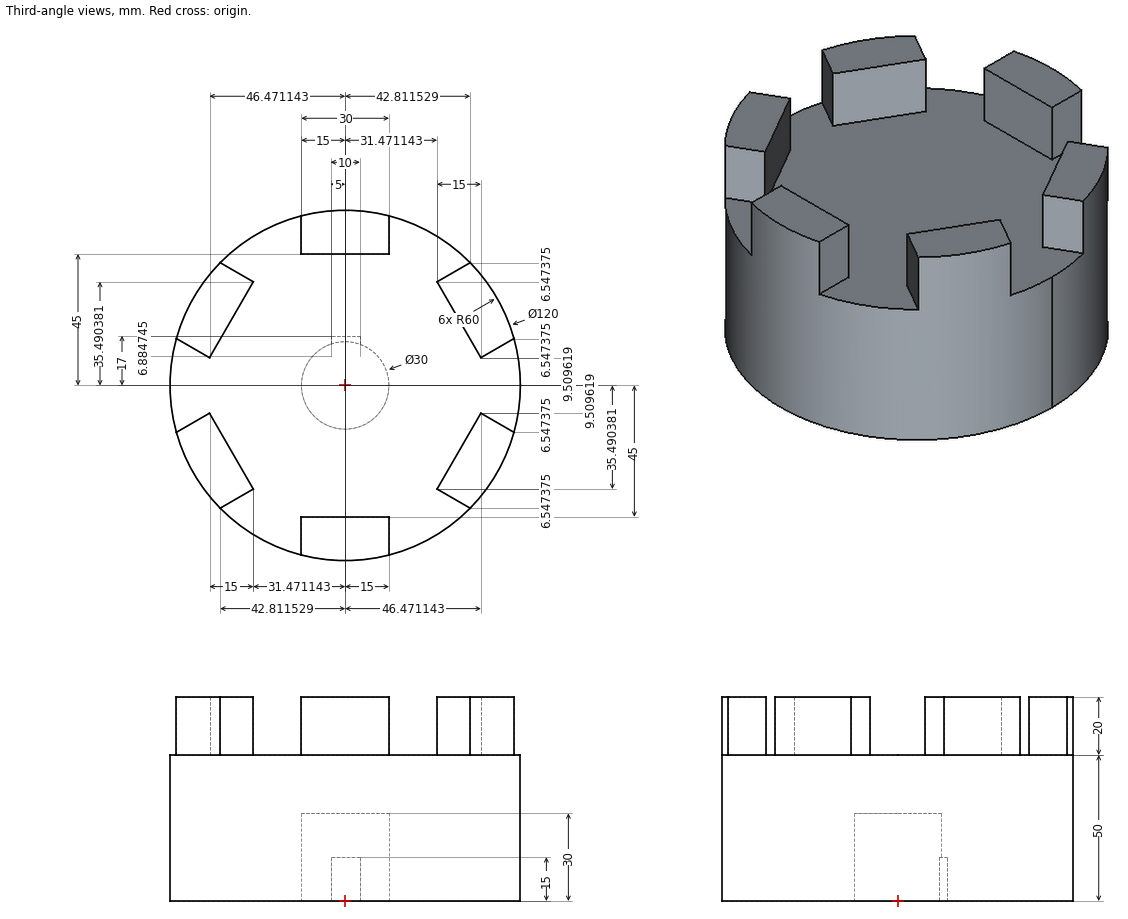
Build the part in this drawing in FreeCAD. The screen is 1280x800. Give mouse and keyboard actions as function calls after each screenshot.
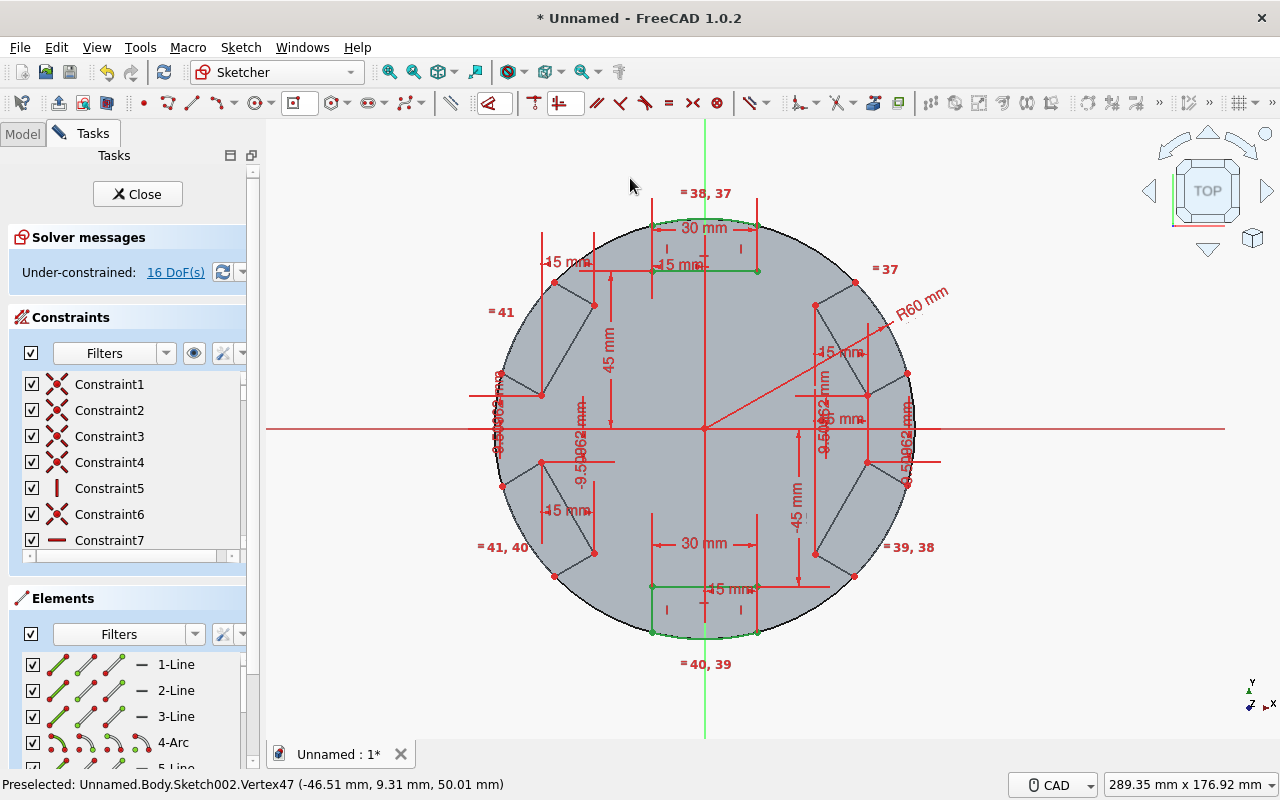
scroll(844, 290, up, 3)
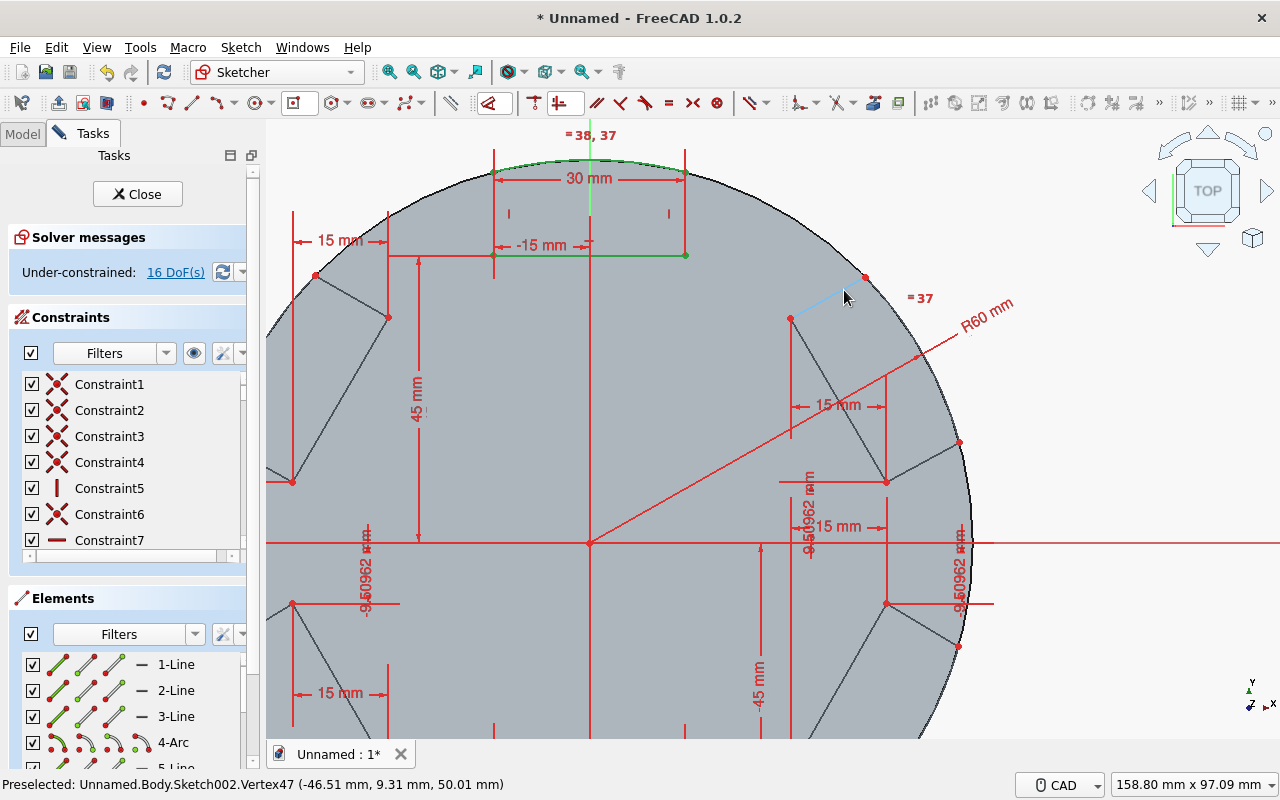
click(843, 290)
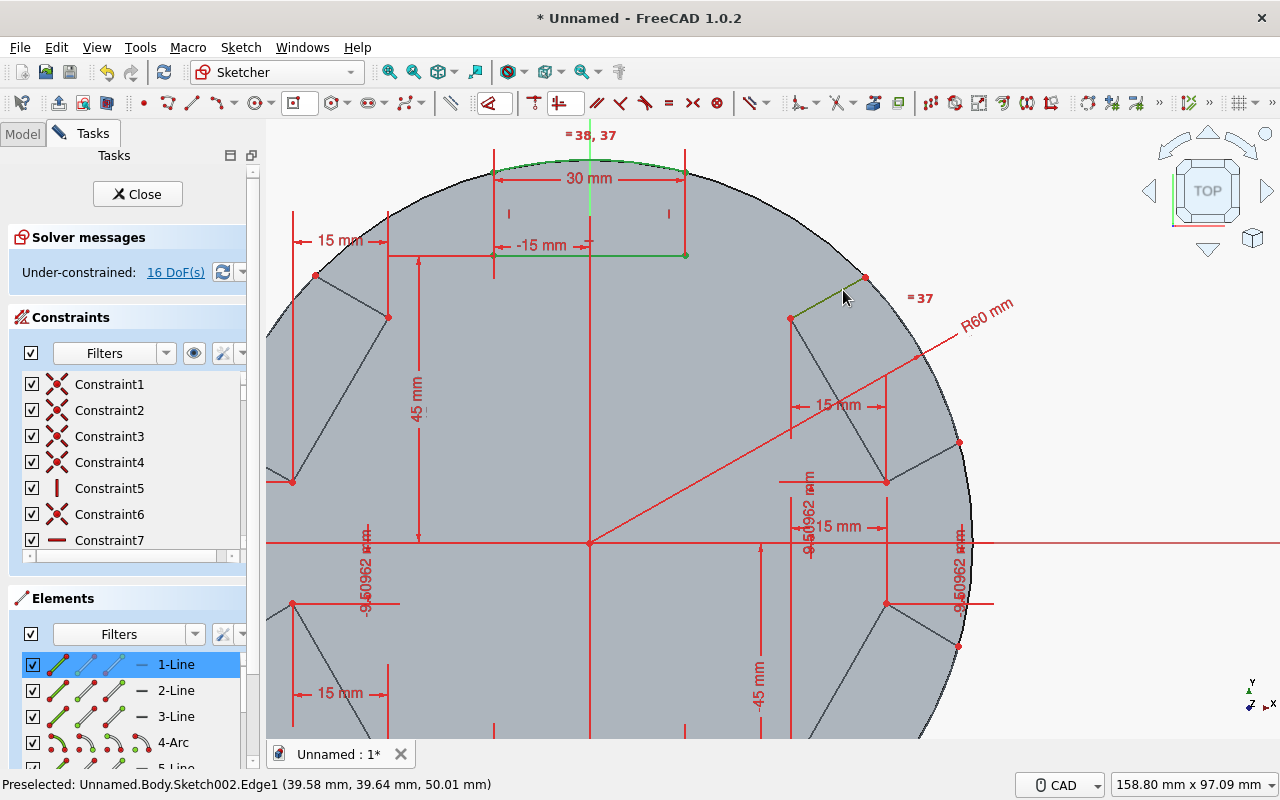
key(i)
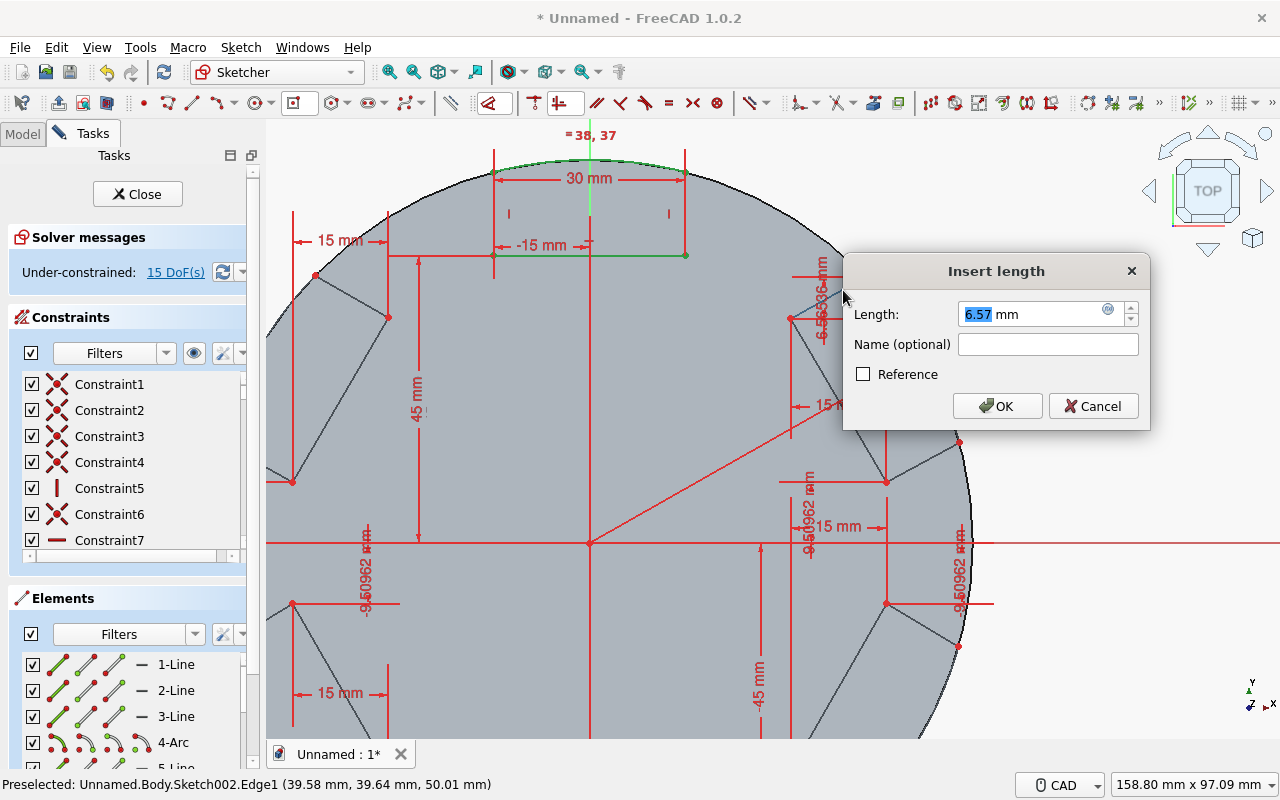
text(6.547375)
key(Return)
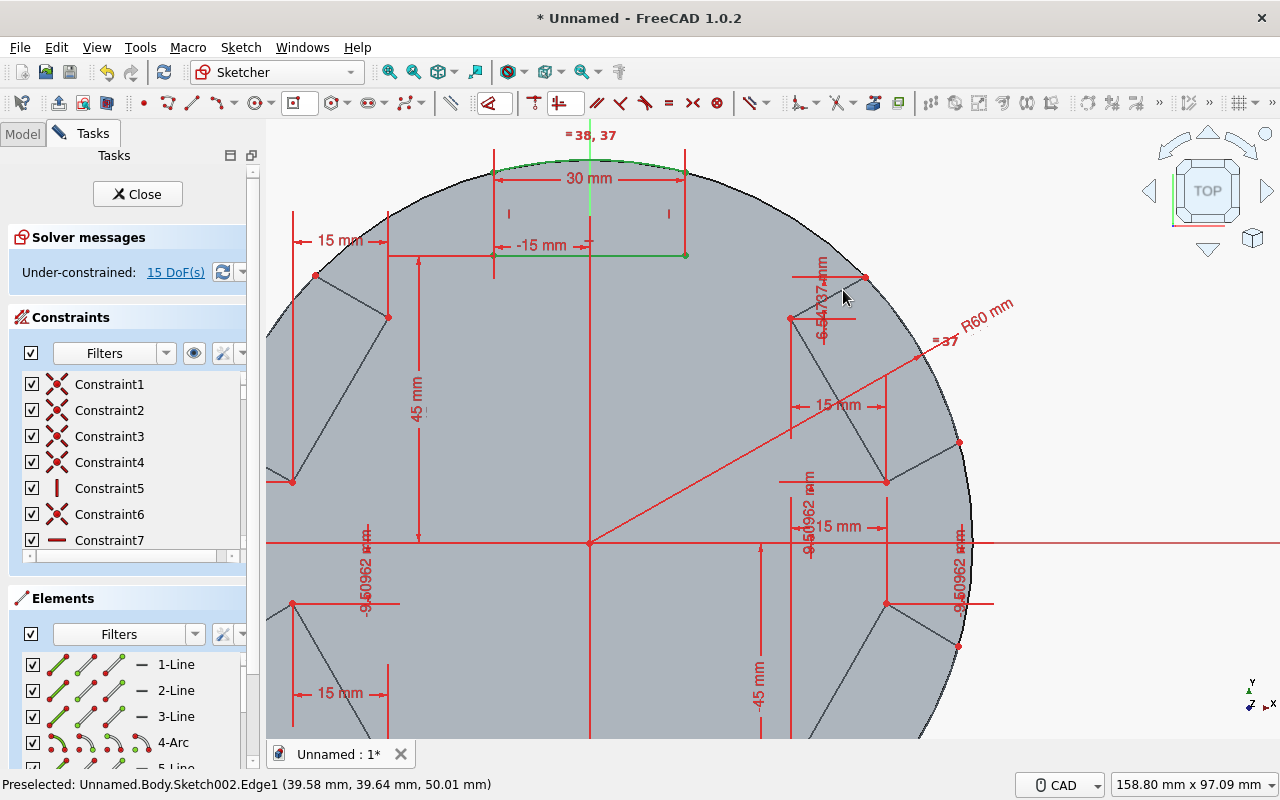
click(908, 470)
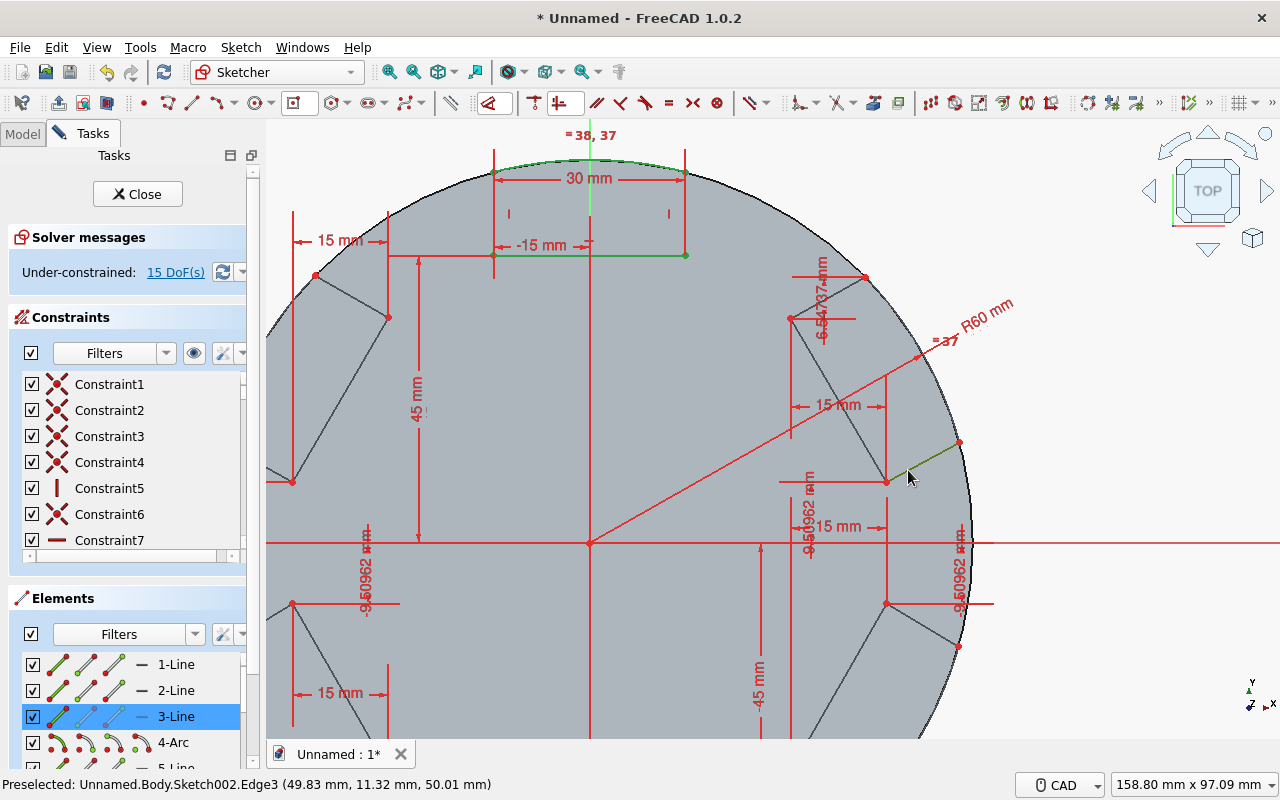
key(i)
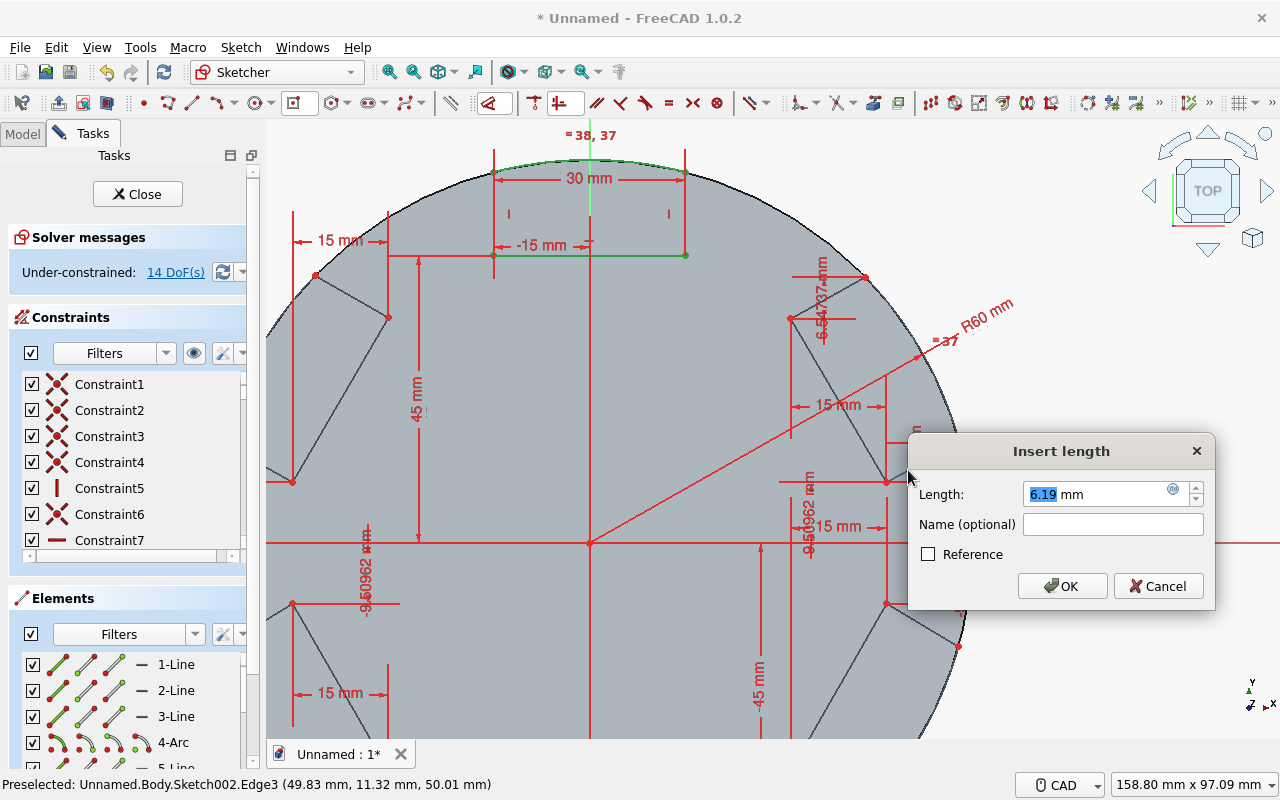
text(6.547375)
key(Return)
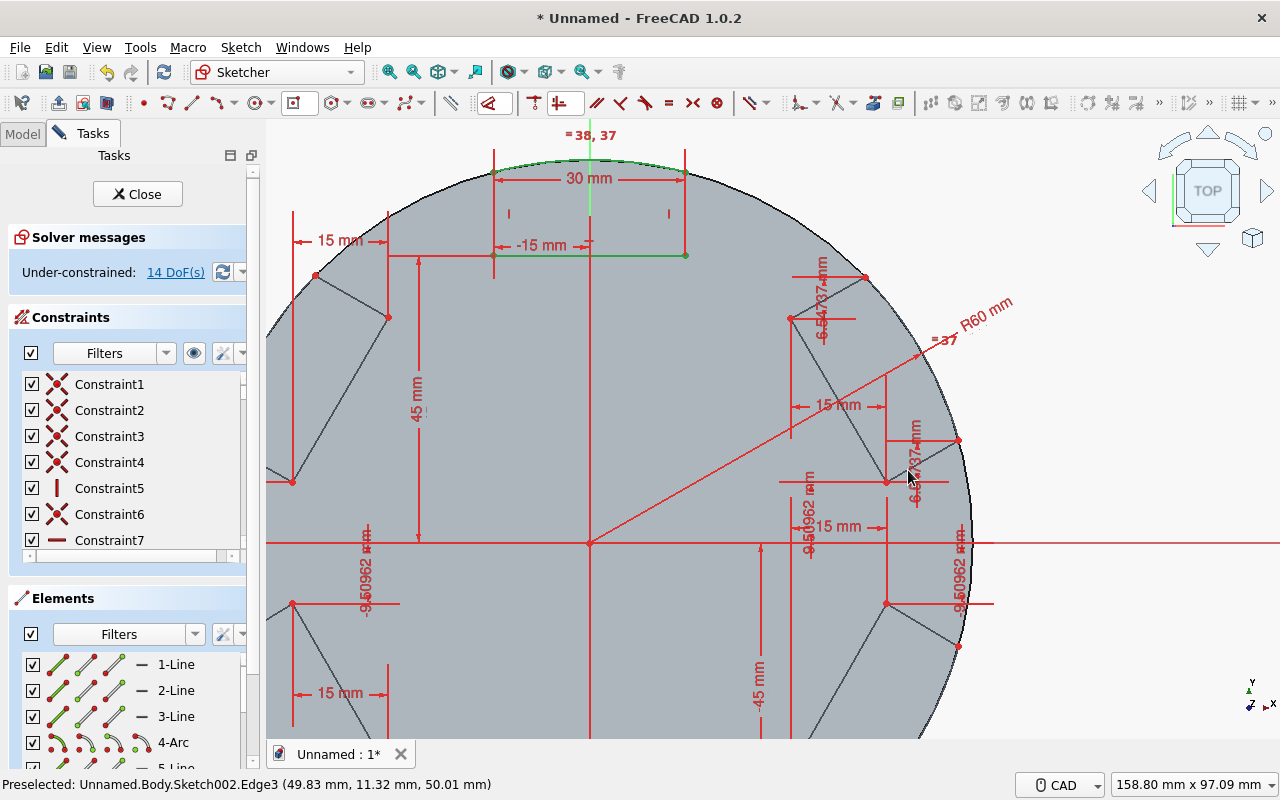
click(937, 634)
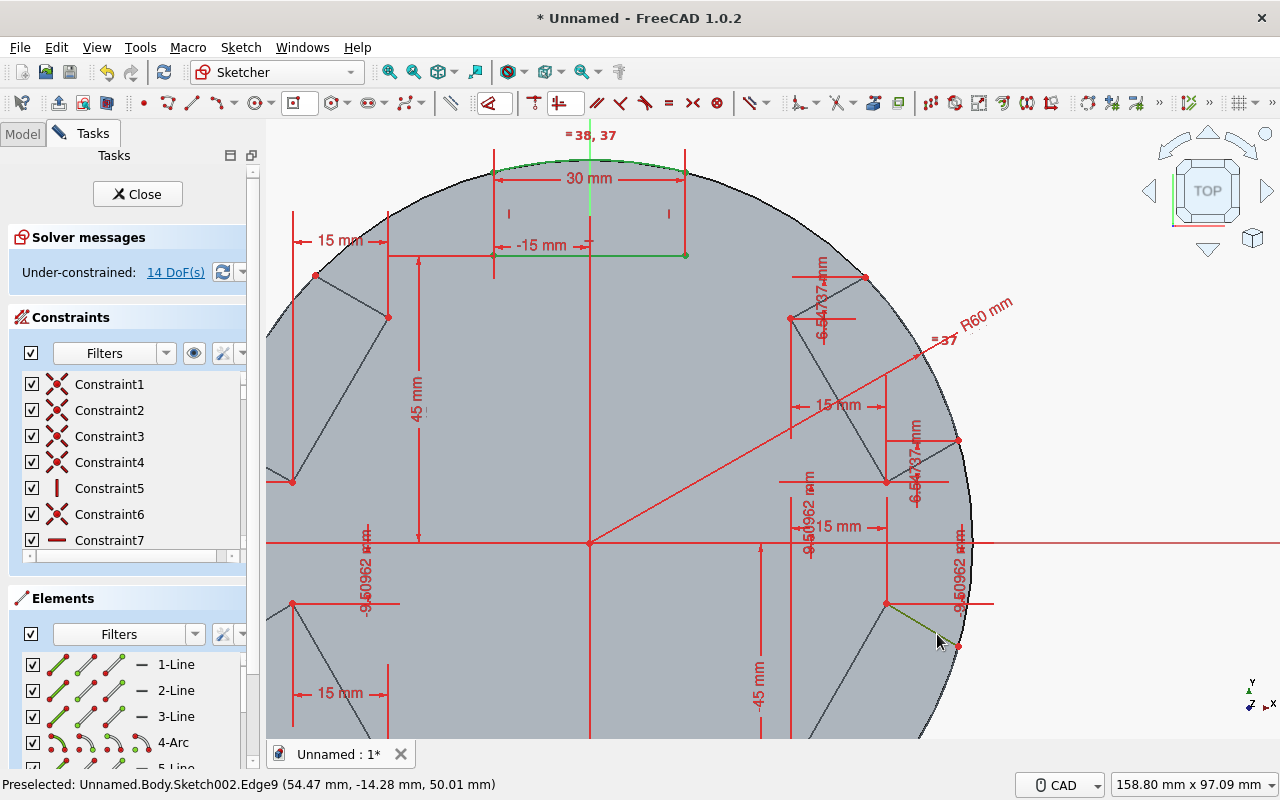
key(i)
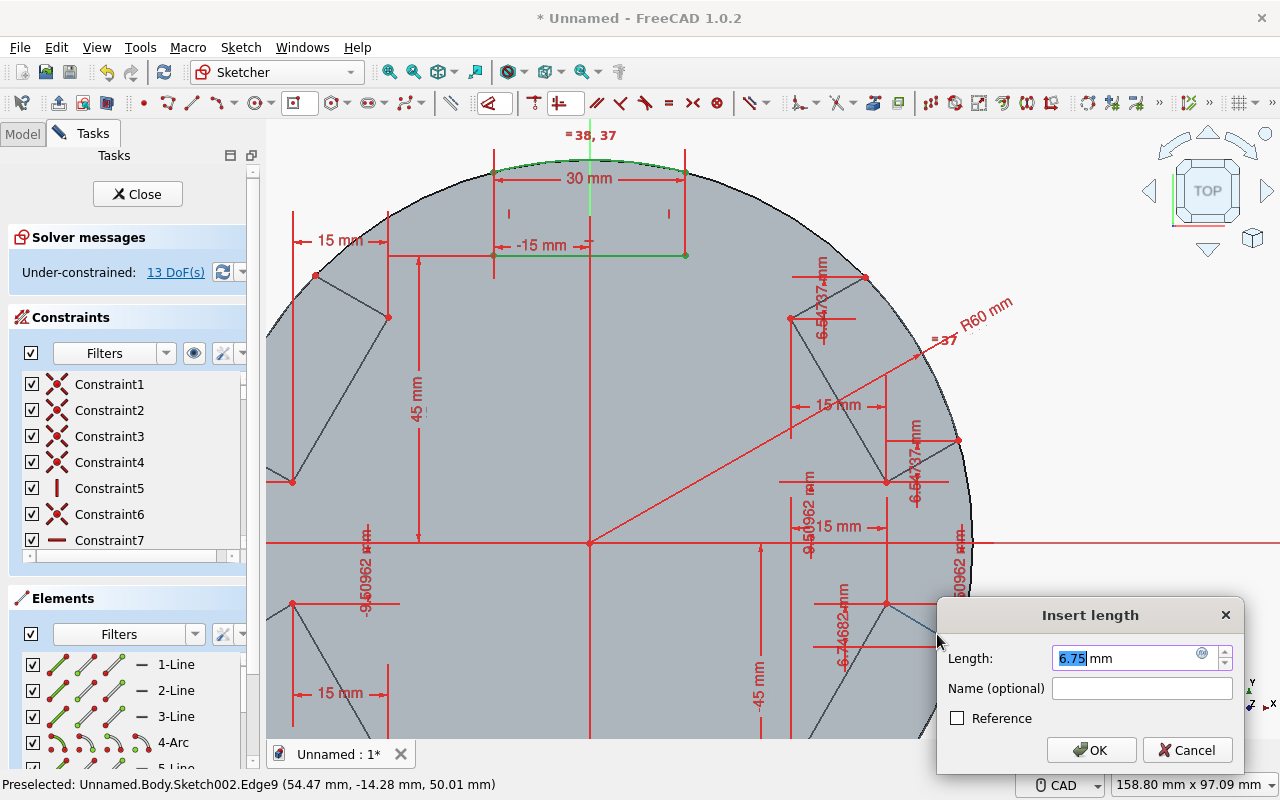
text(6.547375)
key(Return)